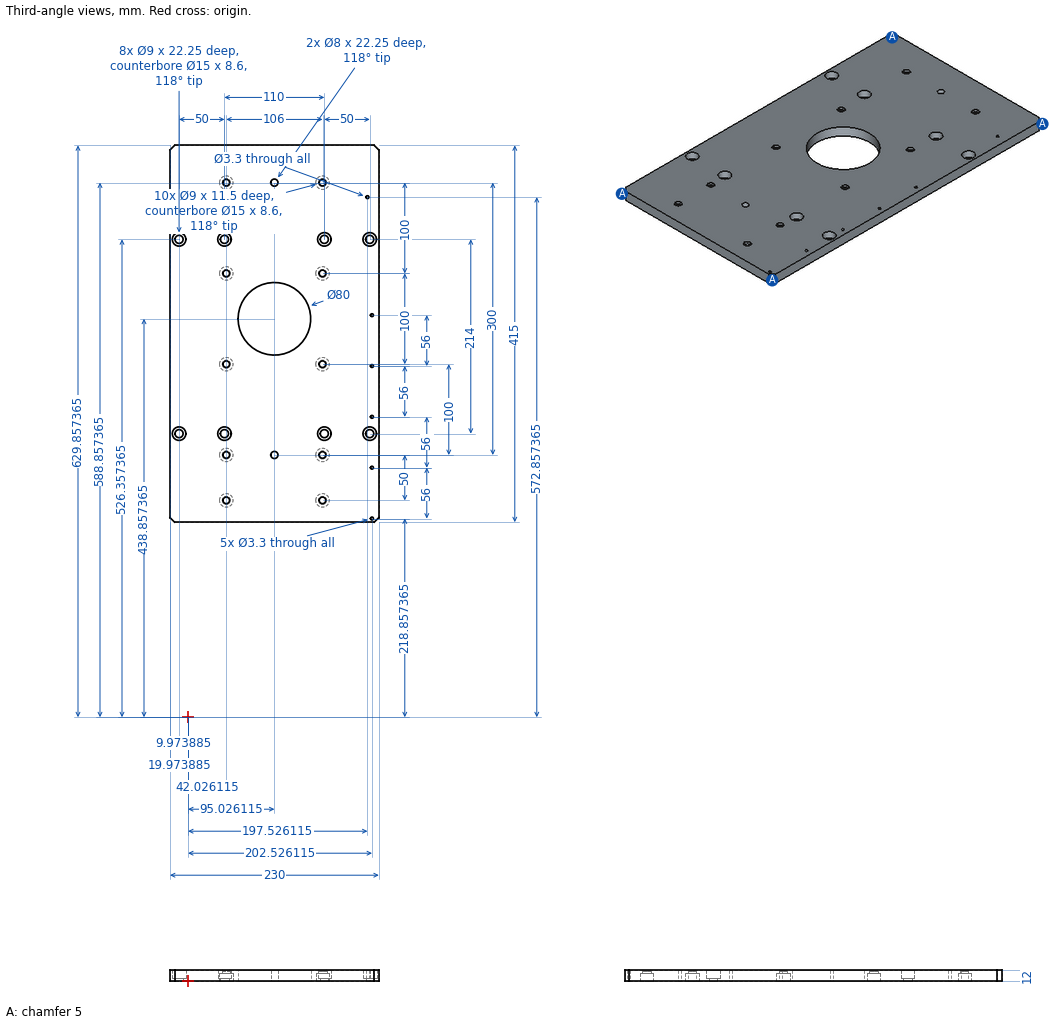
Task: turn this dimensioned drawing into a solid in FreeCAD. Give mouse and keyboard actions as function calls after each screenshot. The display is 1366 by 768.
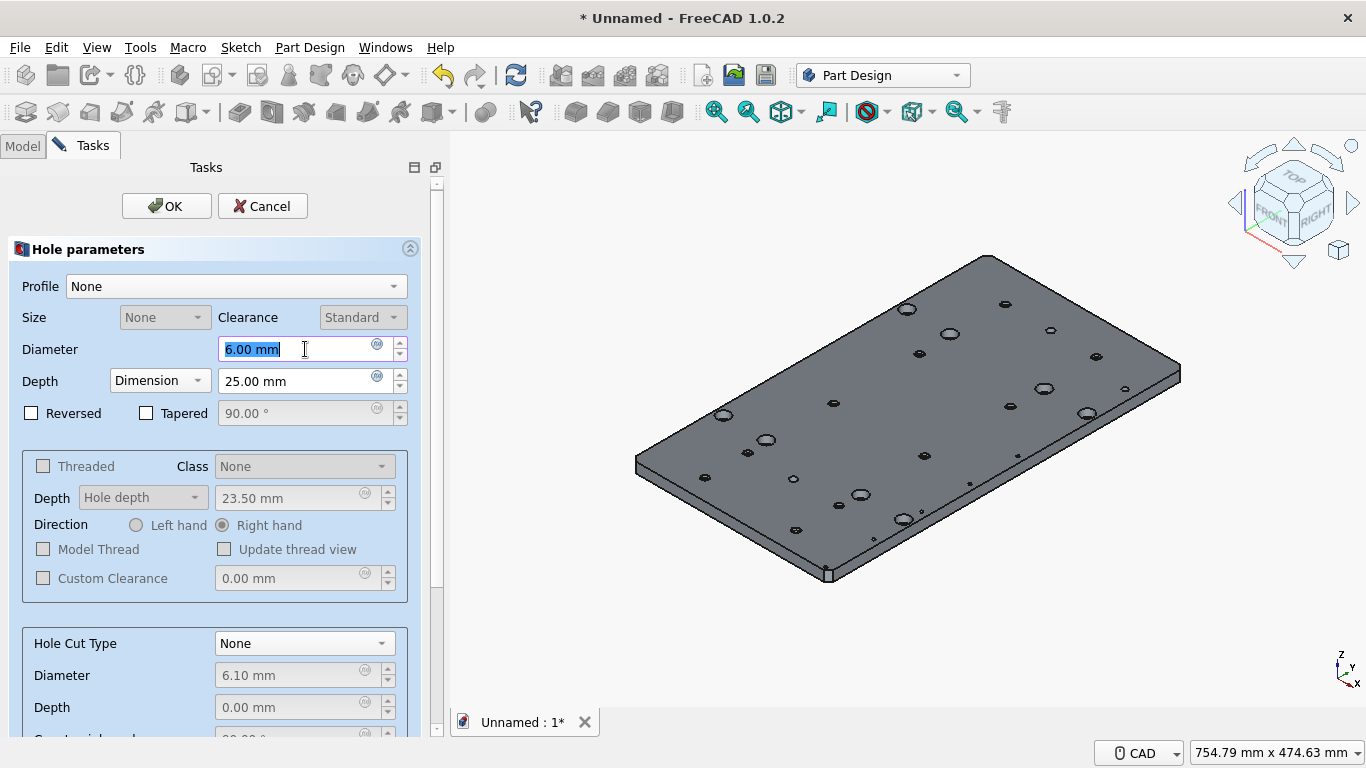
text(3.3)
key(Tab)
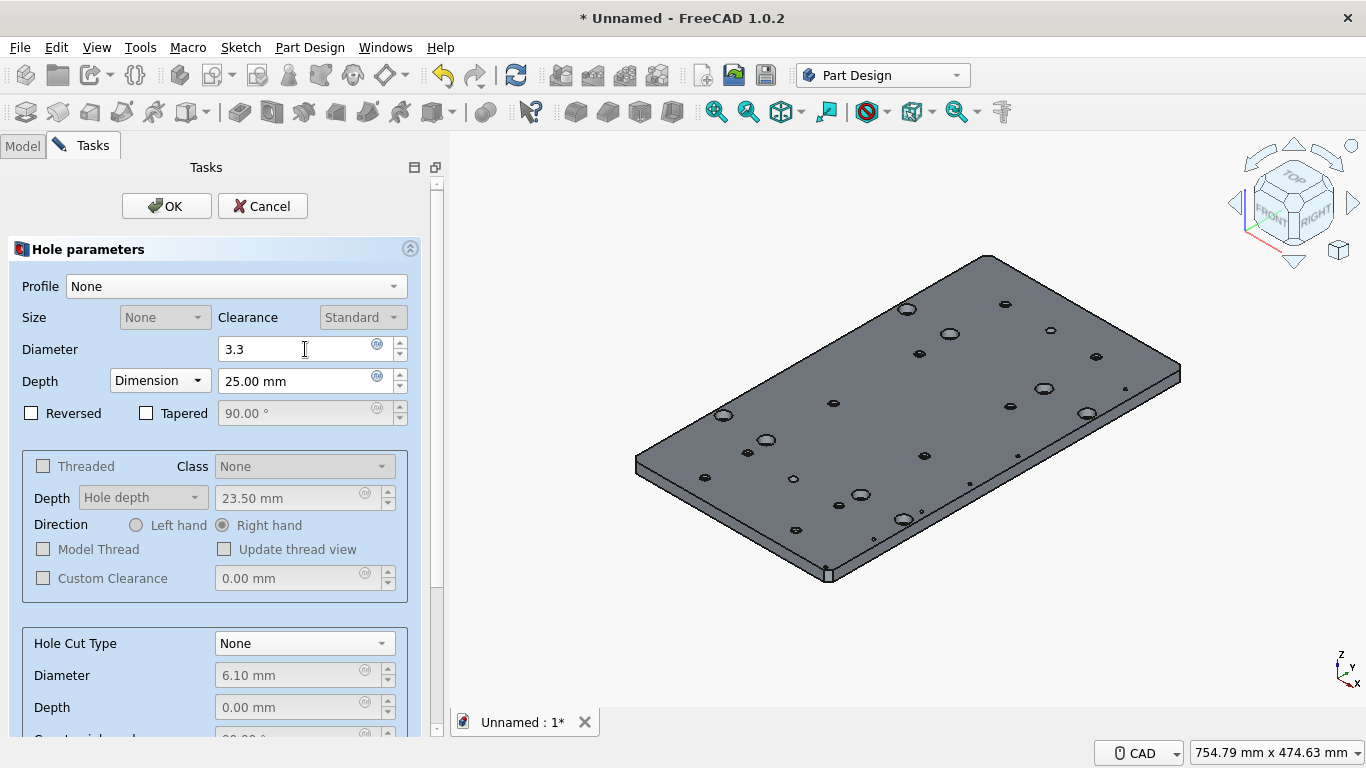
click(161, 380)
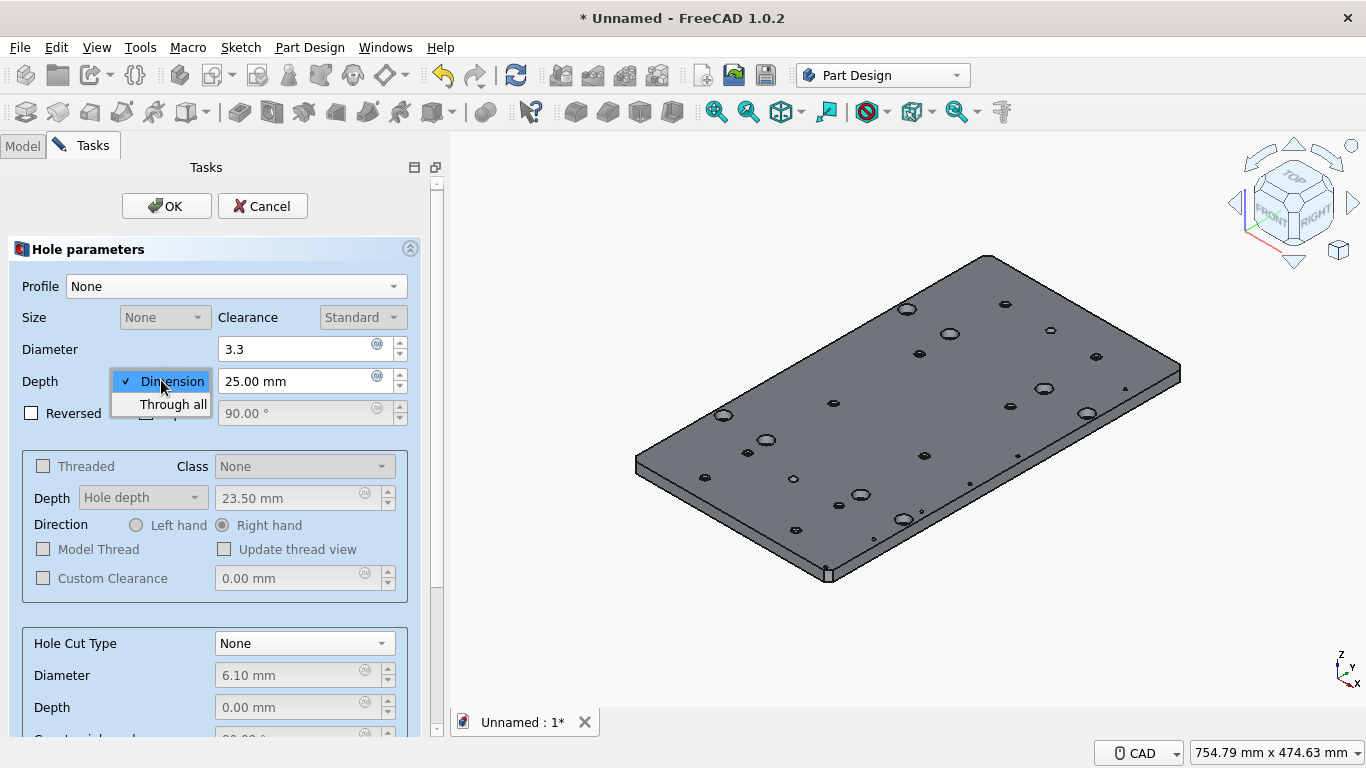
click(160, 404)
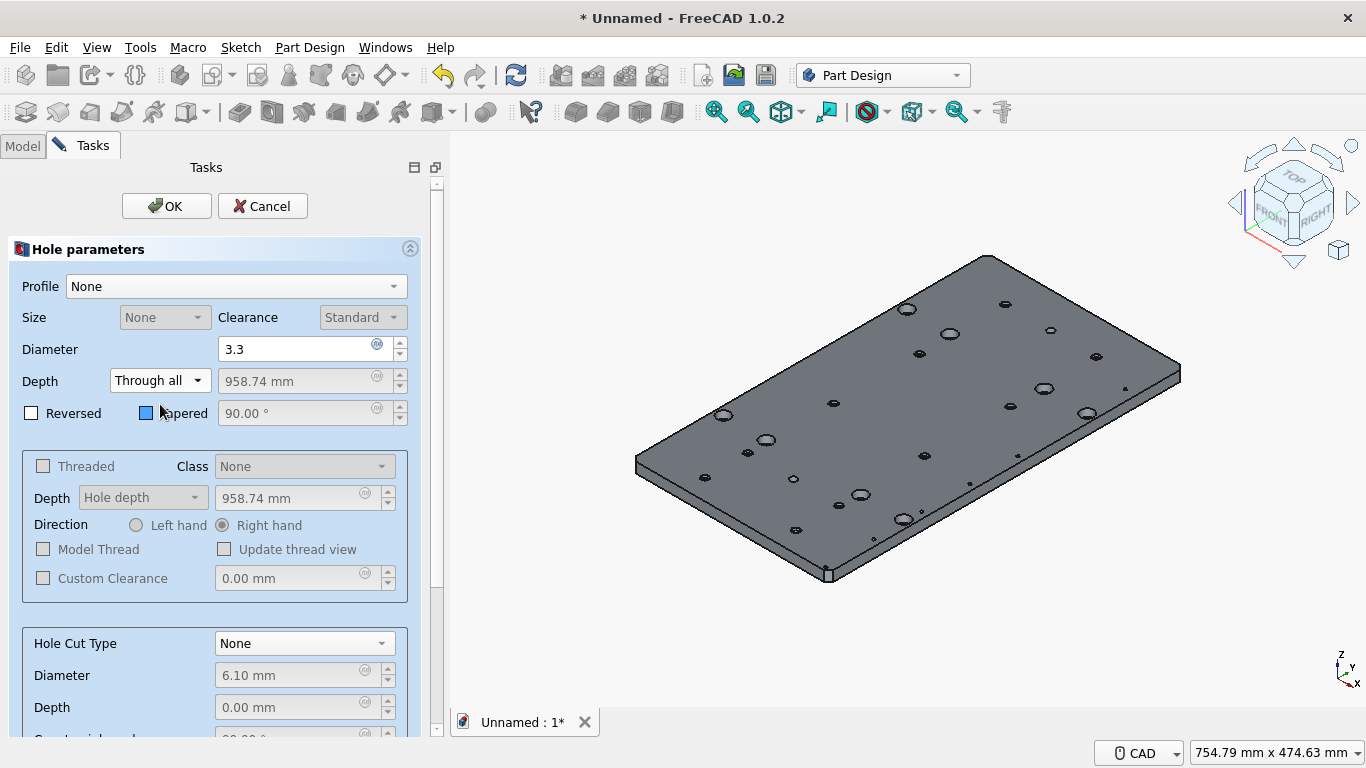
click(167, 206)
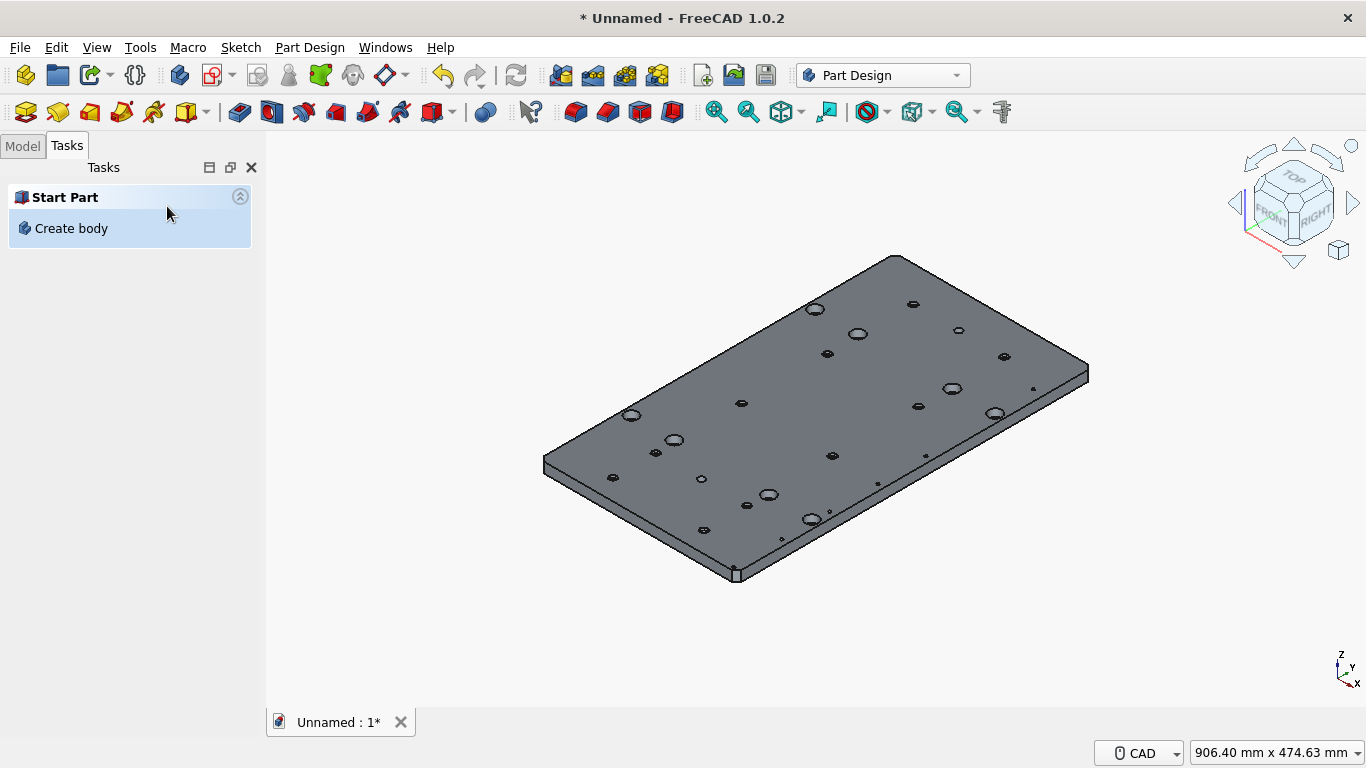
click(212, 76)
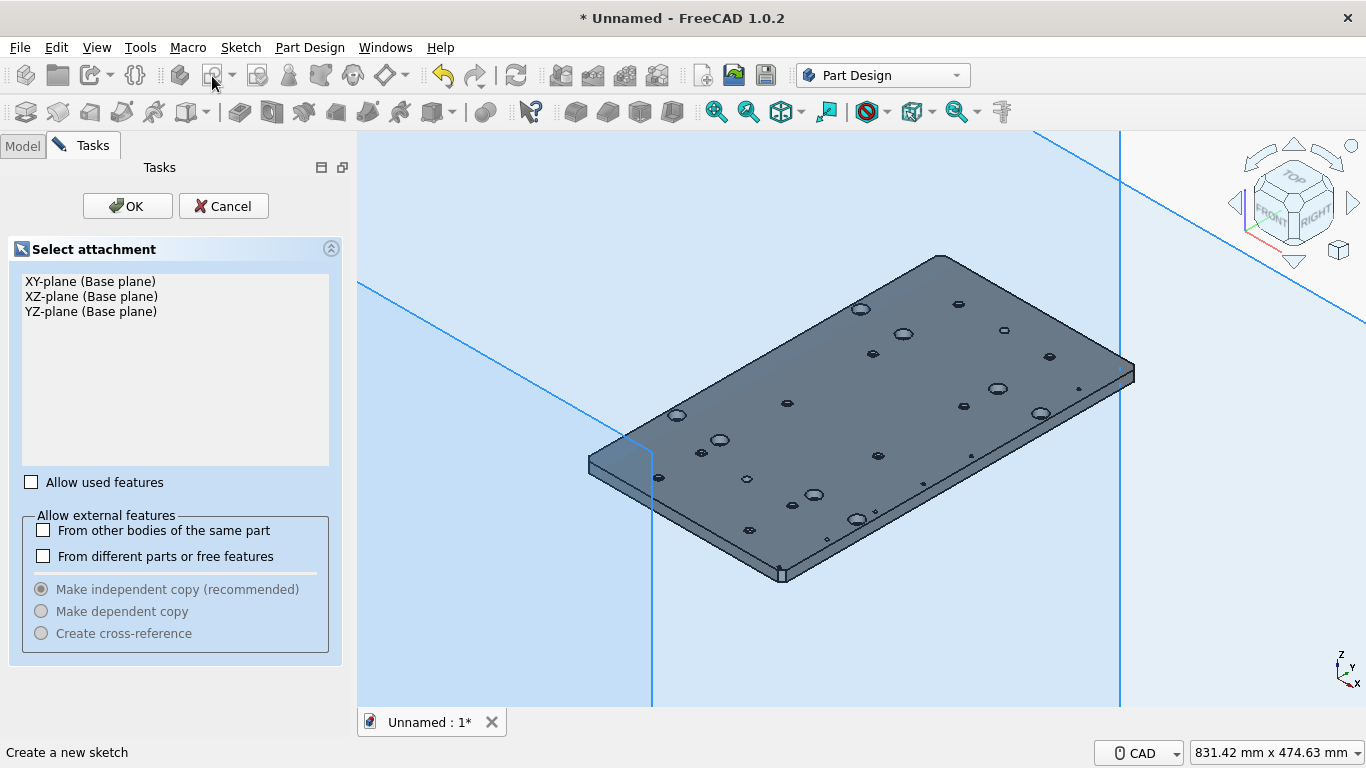
click(82, 282)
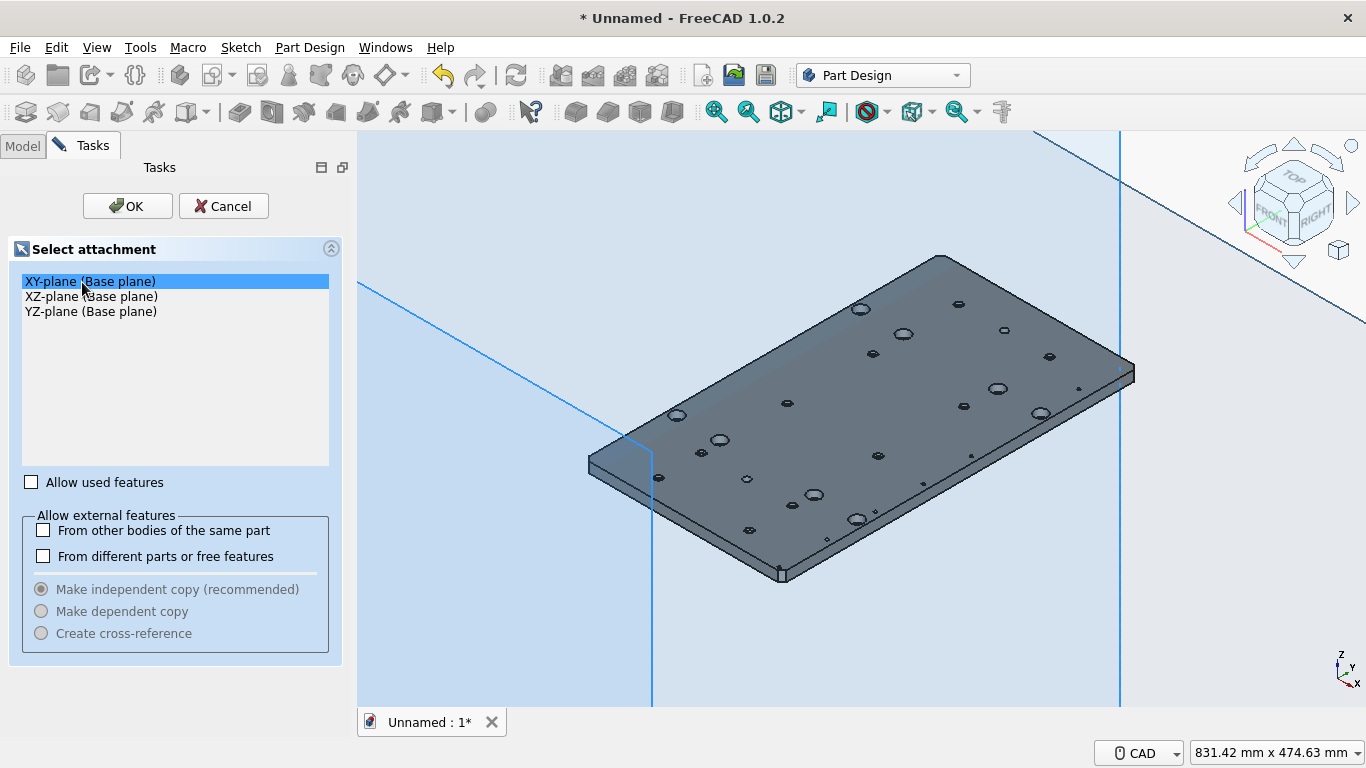
click(128, 206)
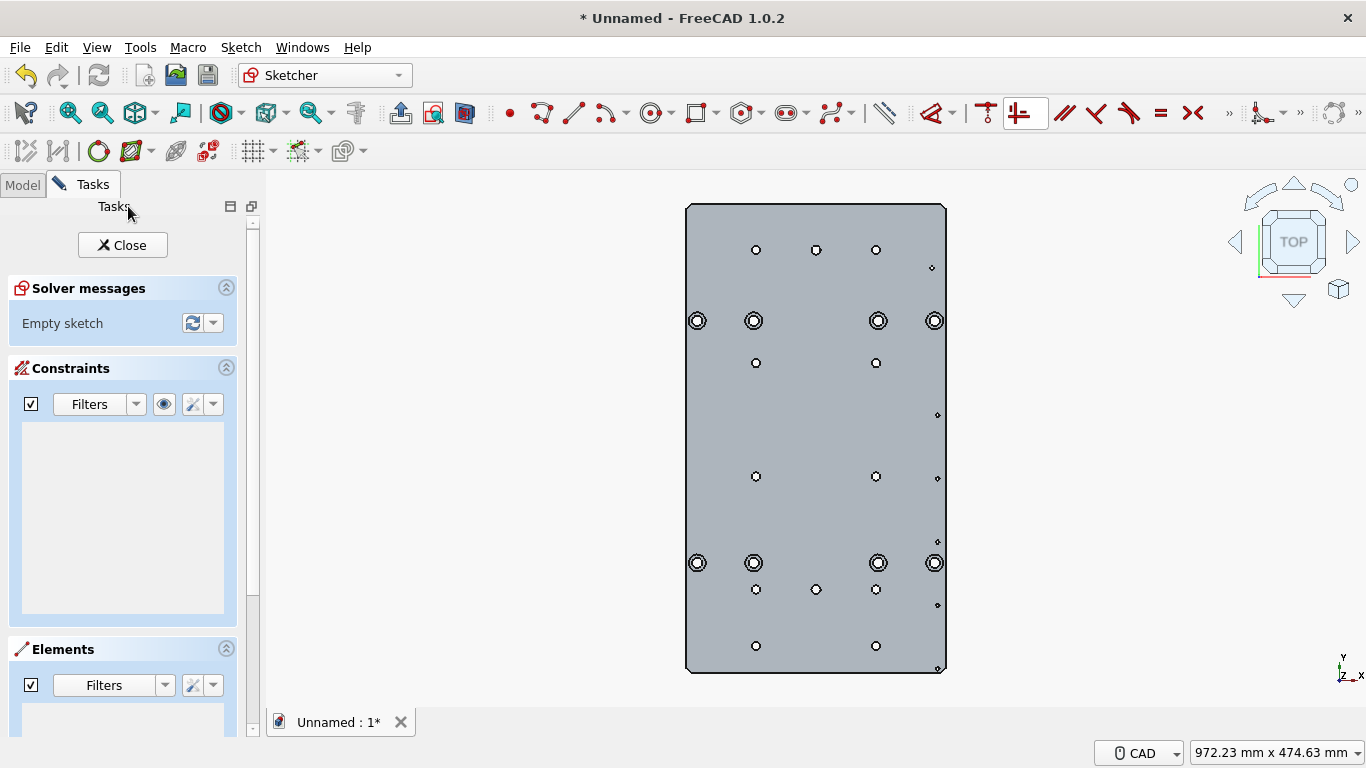
click(466, 114)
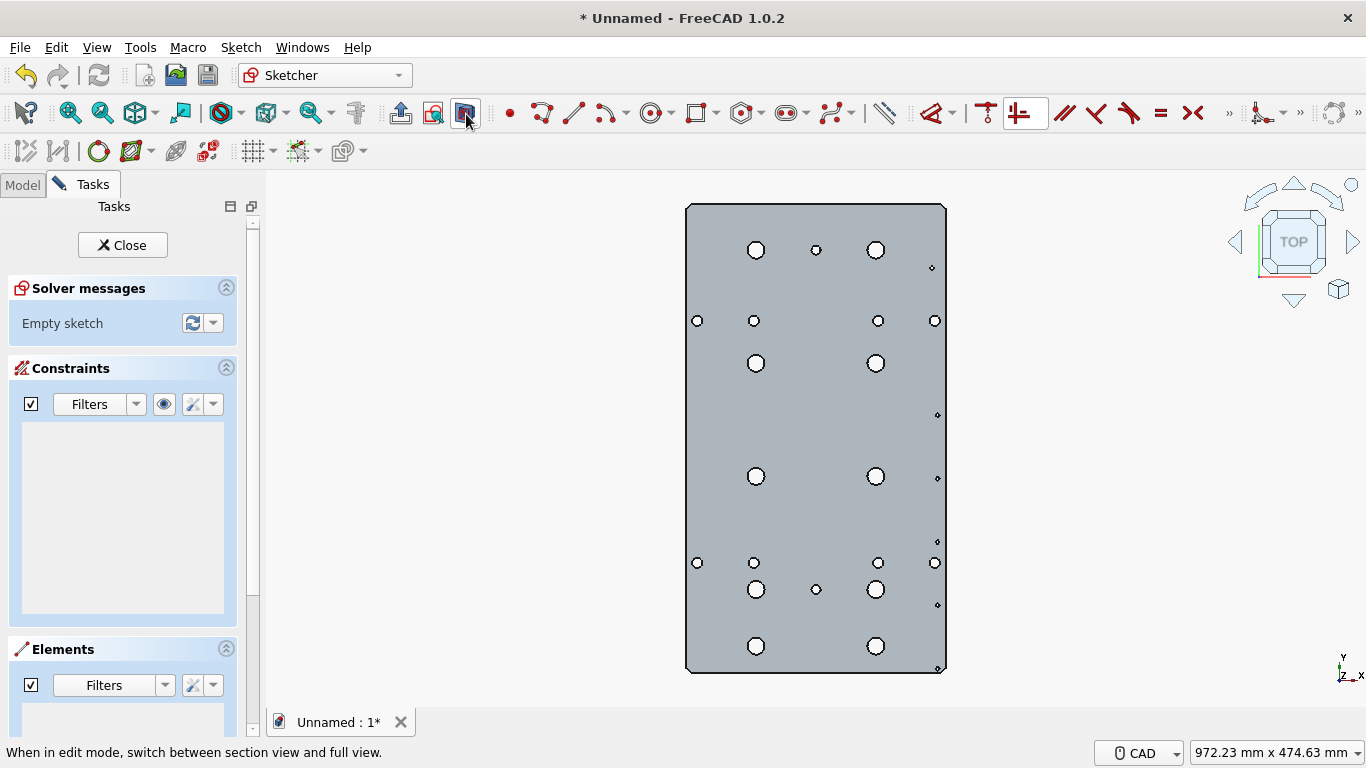
scroll(838, 414, up, 7)